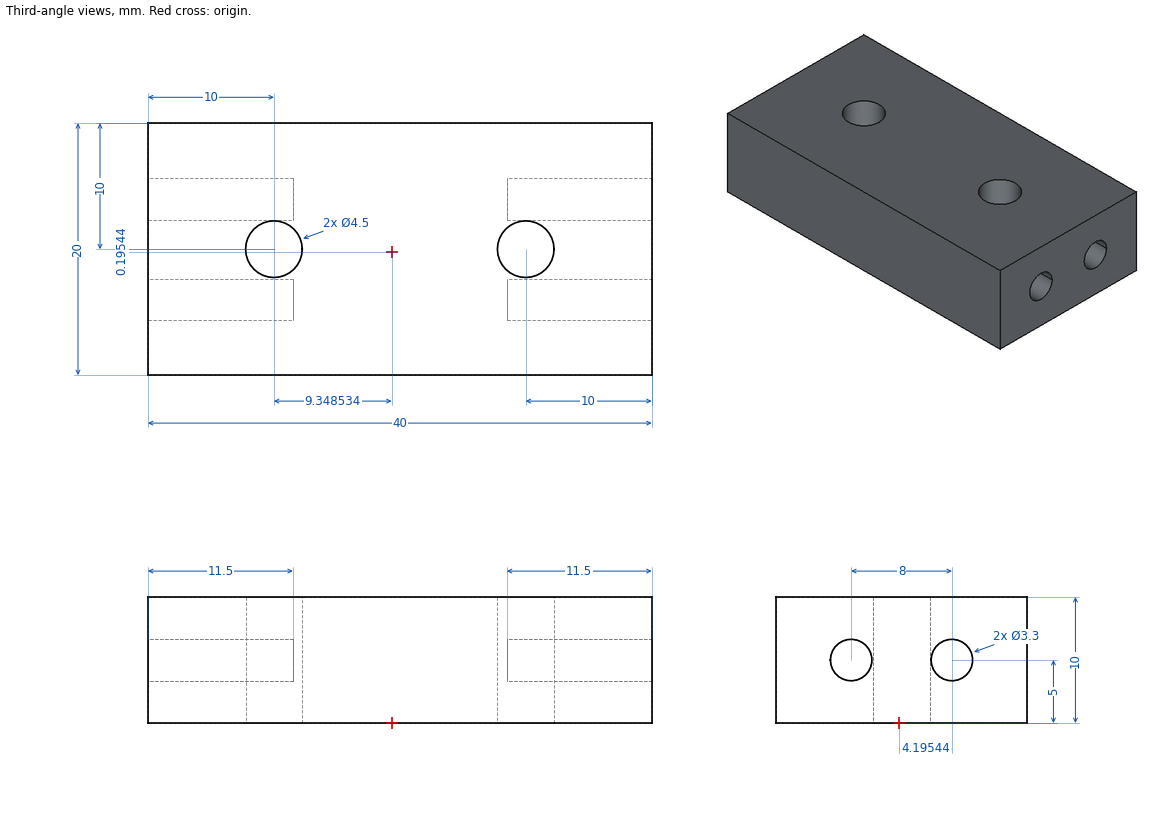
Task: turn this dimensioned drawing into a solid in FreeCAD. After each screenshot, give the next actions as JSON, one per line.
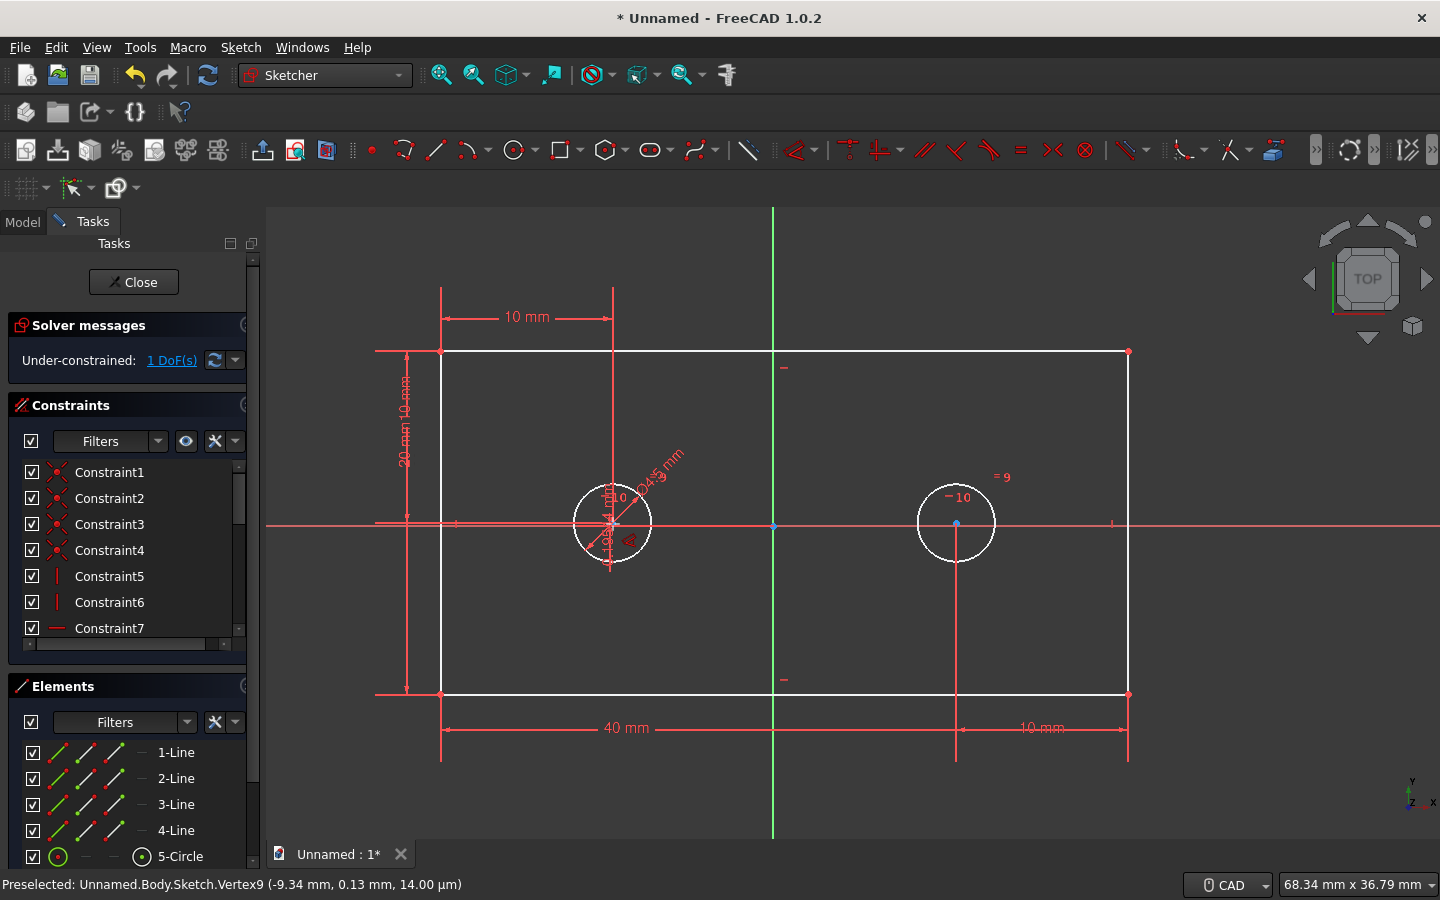
{"action": "left_click", "coordinate": [613, 523]}
{"action": "left_click", "coordinate": [693, 560]}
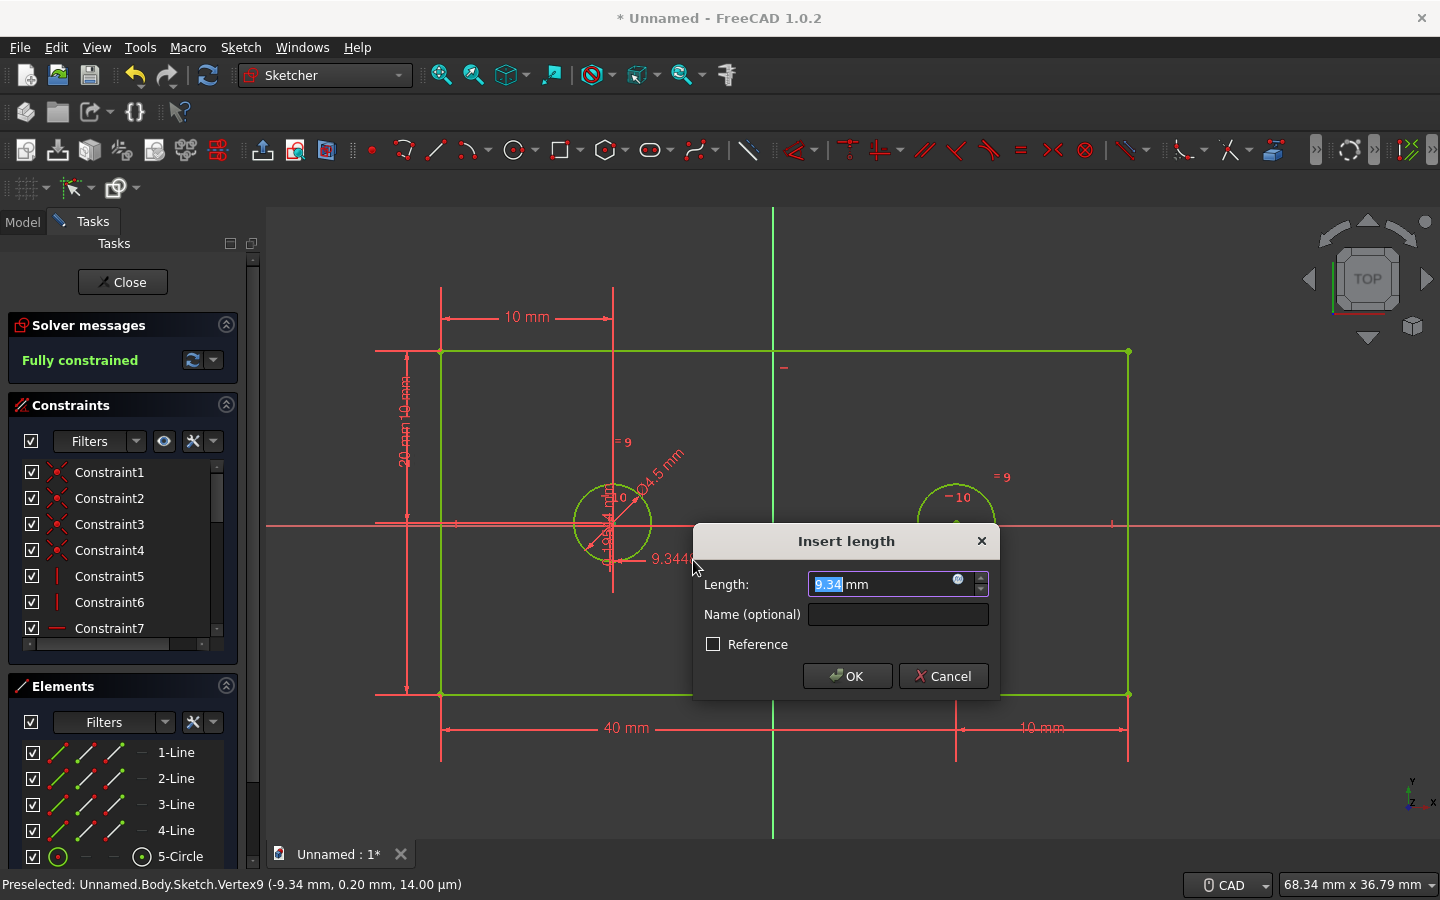
{"action": "type", "text": "9.348534"}
{"action": "key", "text": "Return"}
{"action": "key", "text": "Escape"}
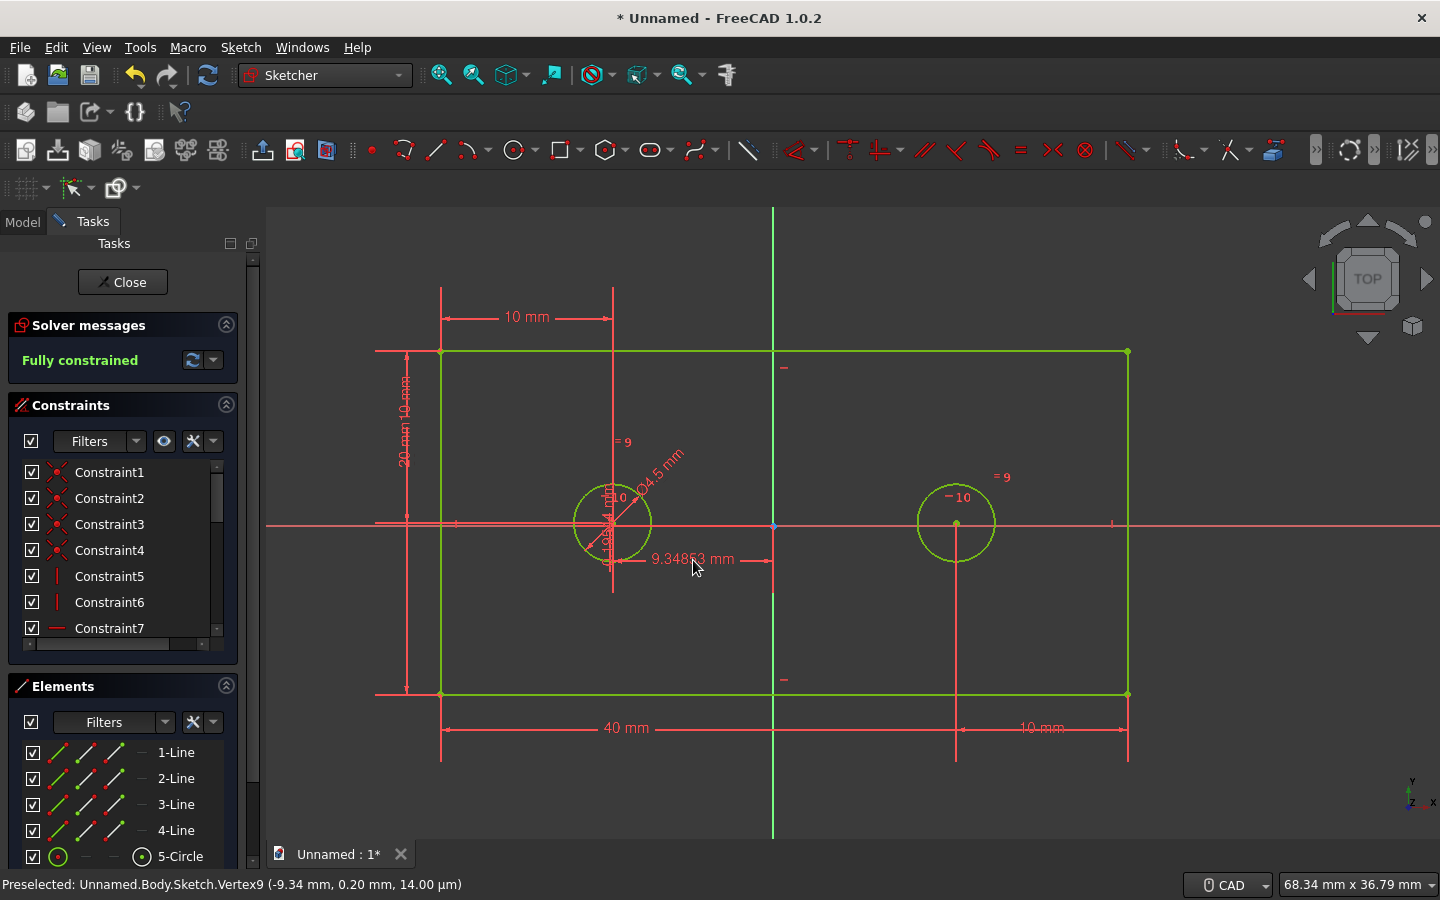
{"action": "left_click", "coordinate": [123, 282]}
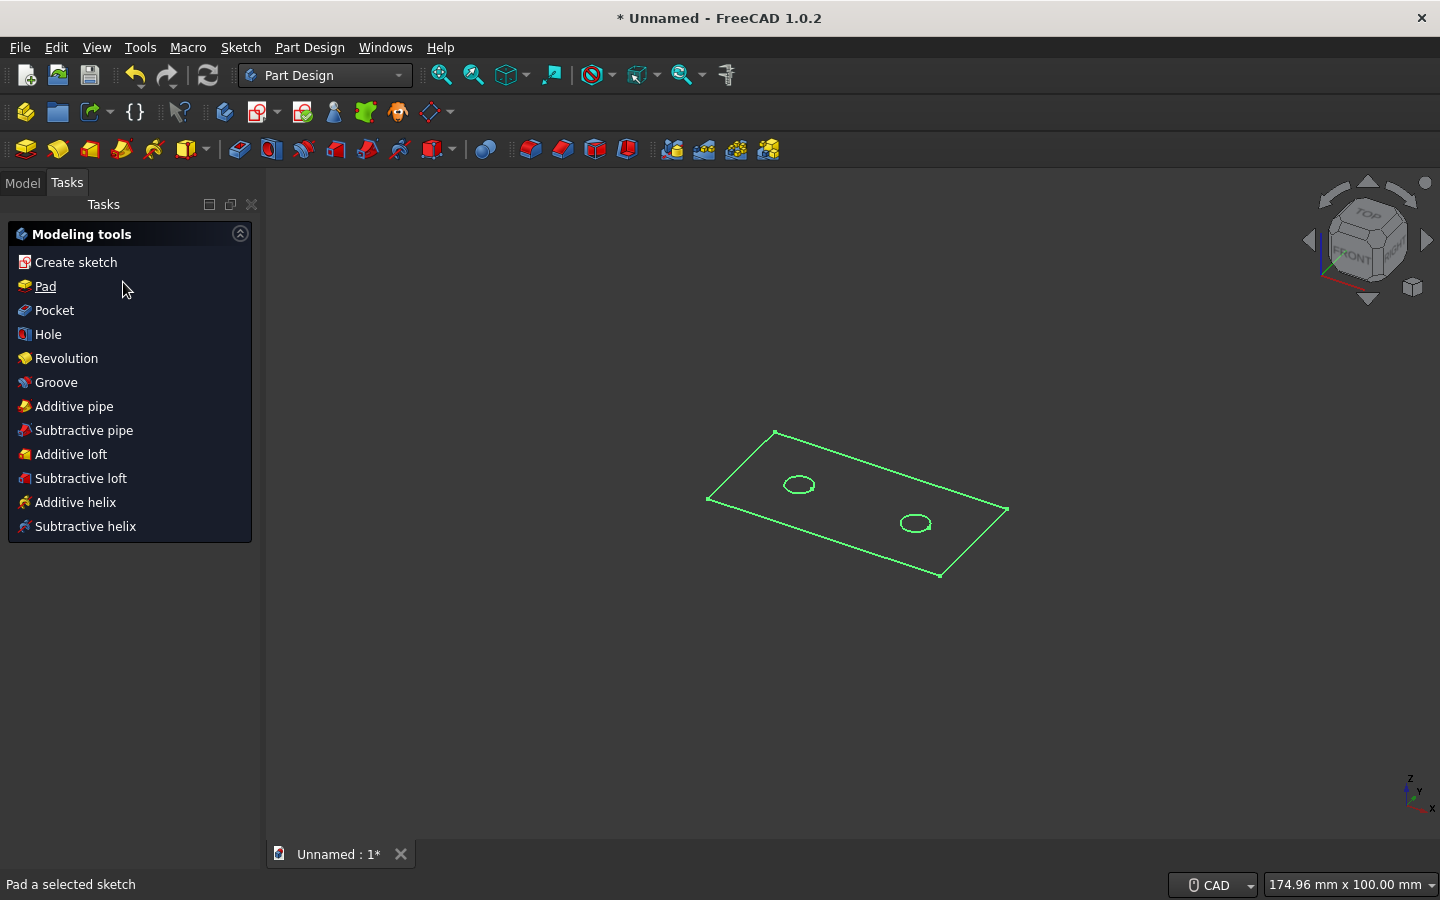
{"action": "left_click", "coordinate": [26, 150]}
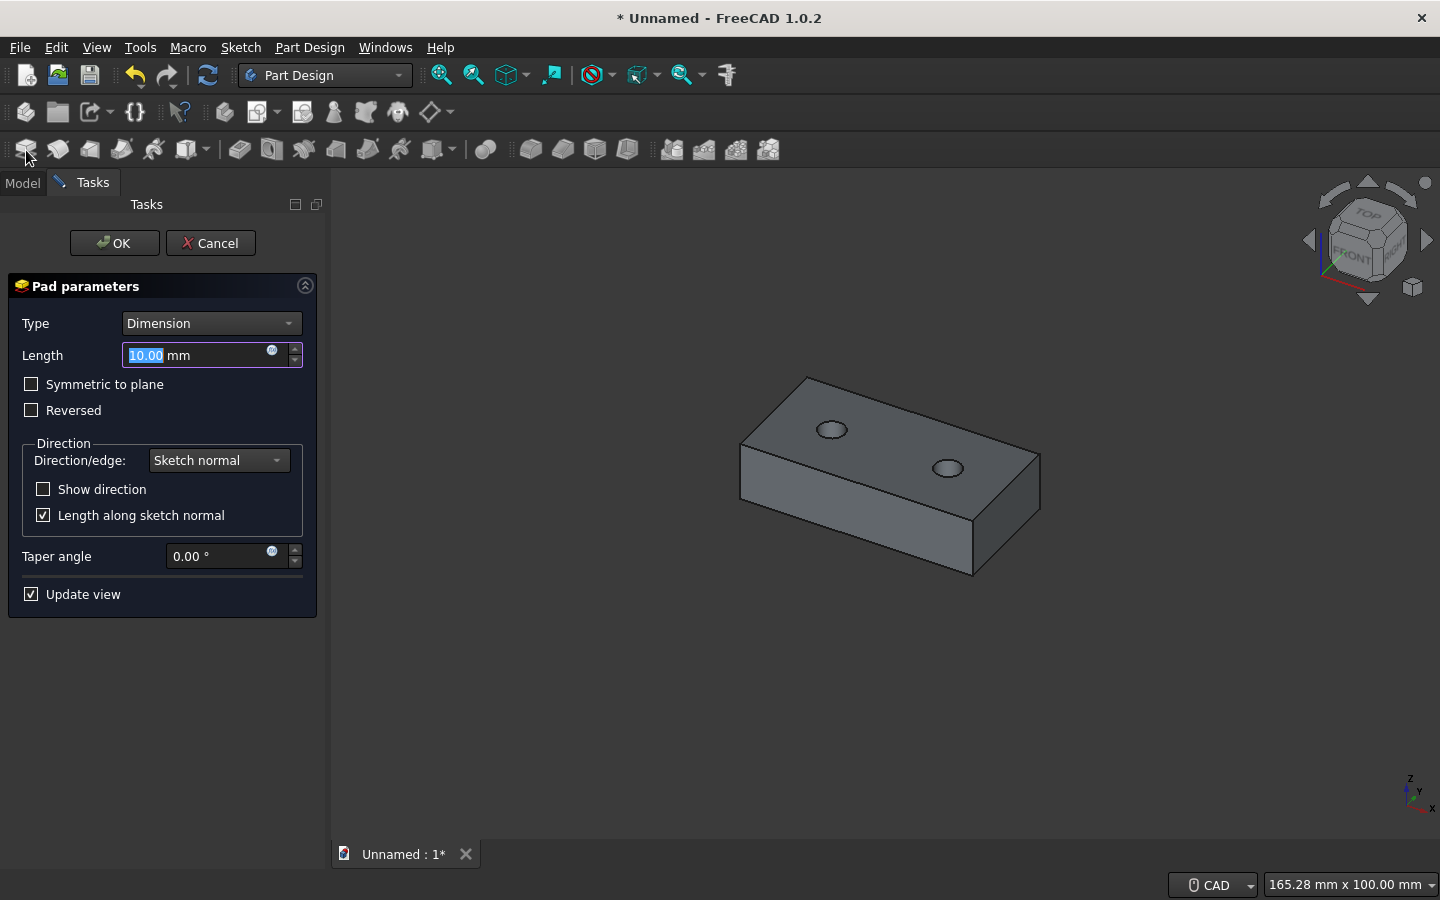
{"action": "type", "text": "10"}
{"action": "key", "text": "Tab"}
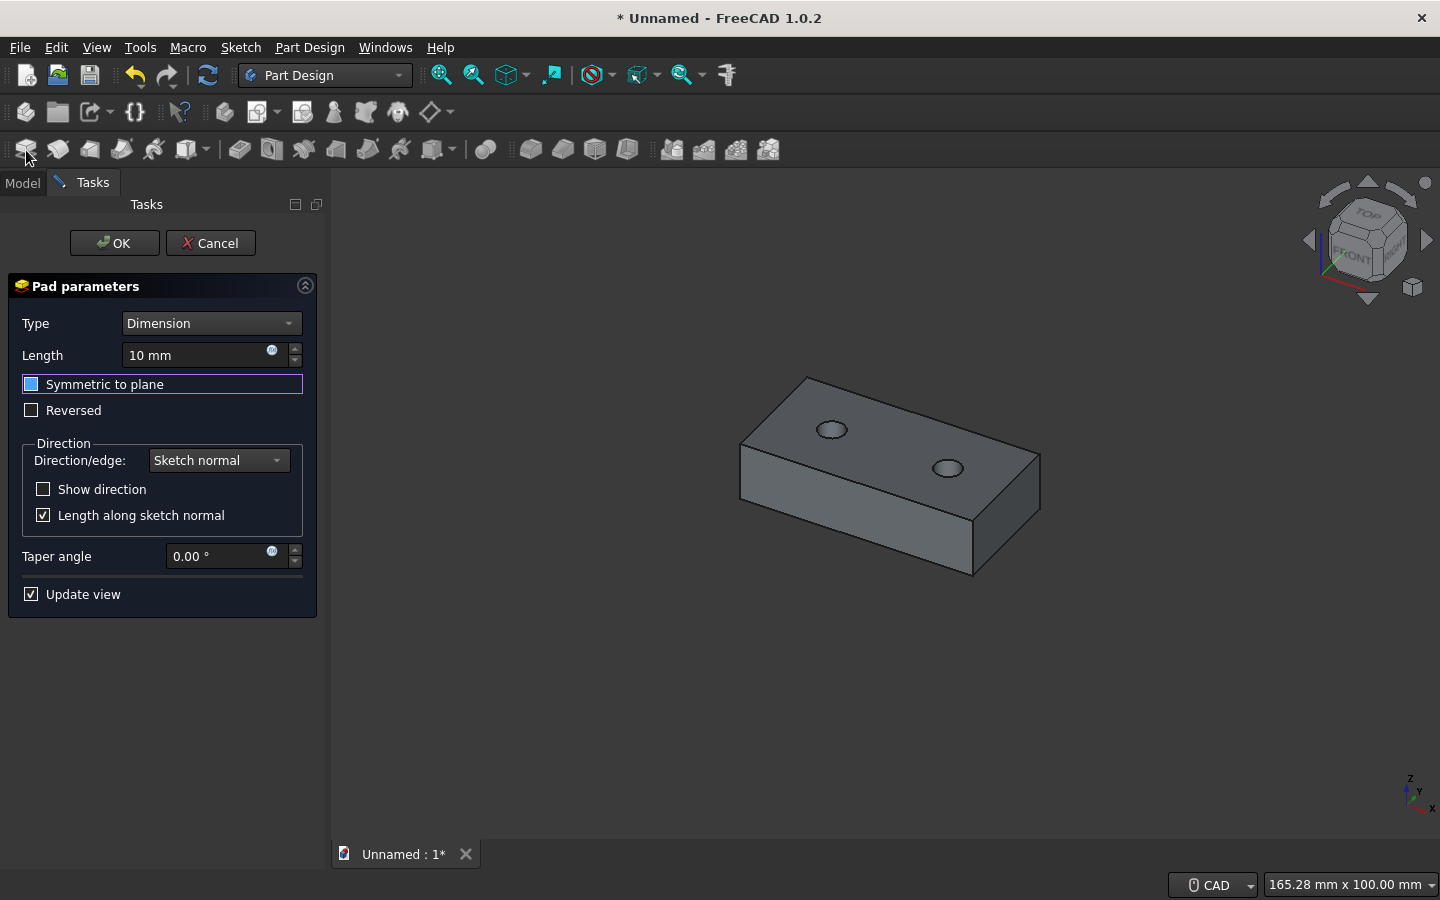
{"action": "left_click", "coordinate": [115, 243]}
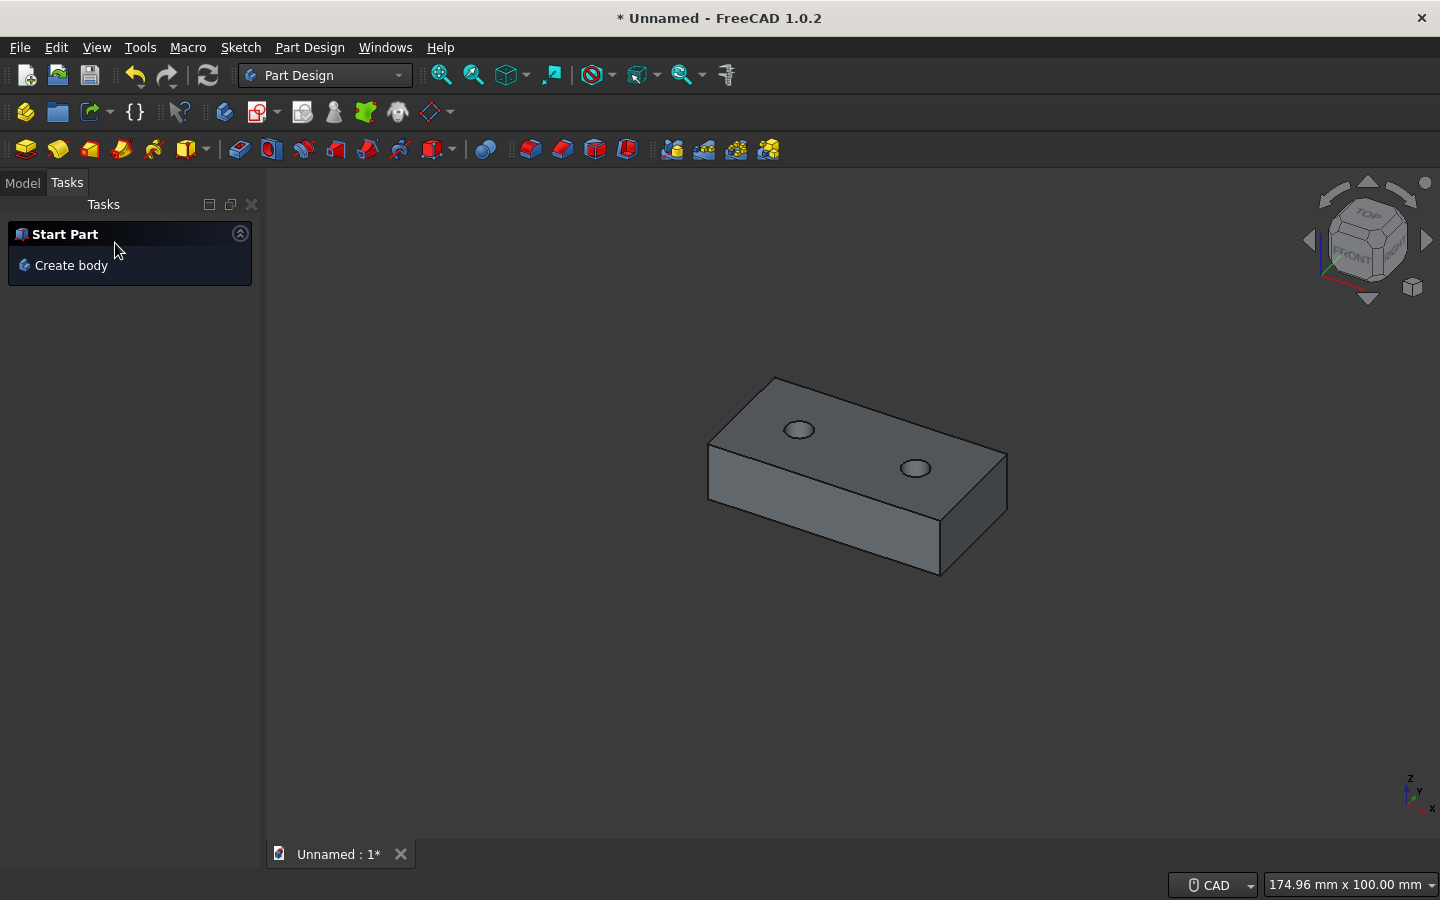
{"action": "key", "text": "v f"}